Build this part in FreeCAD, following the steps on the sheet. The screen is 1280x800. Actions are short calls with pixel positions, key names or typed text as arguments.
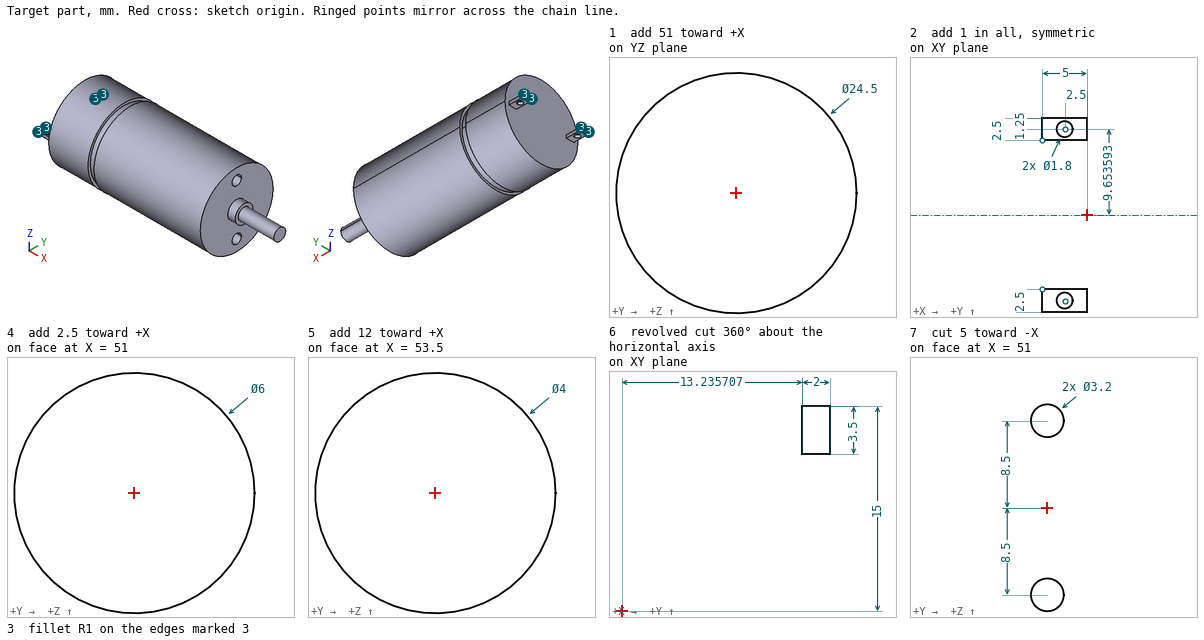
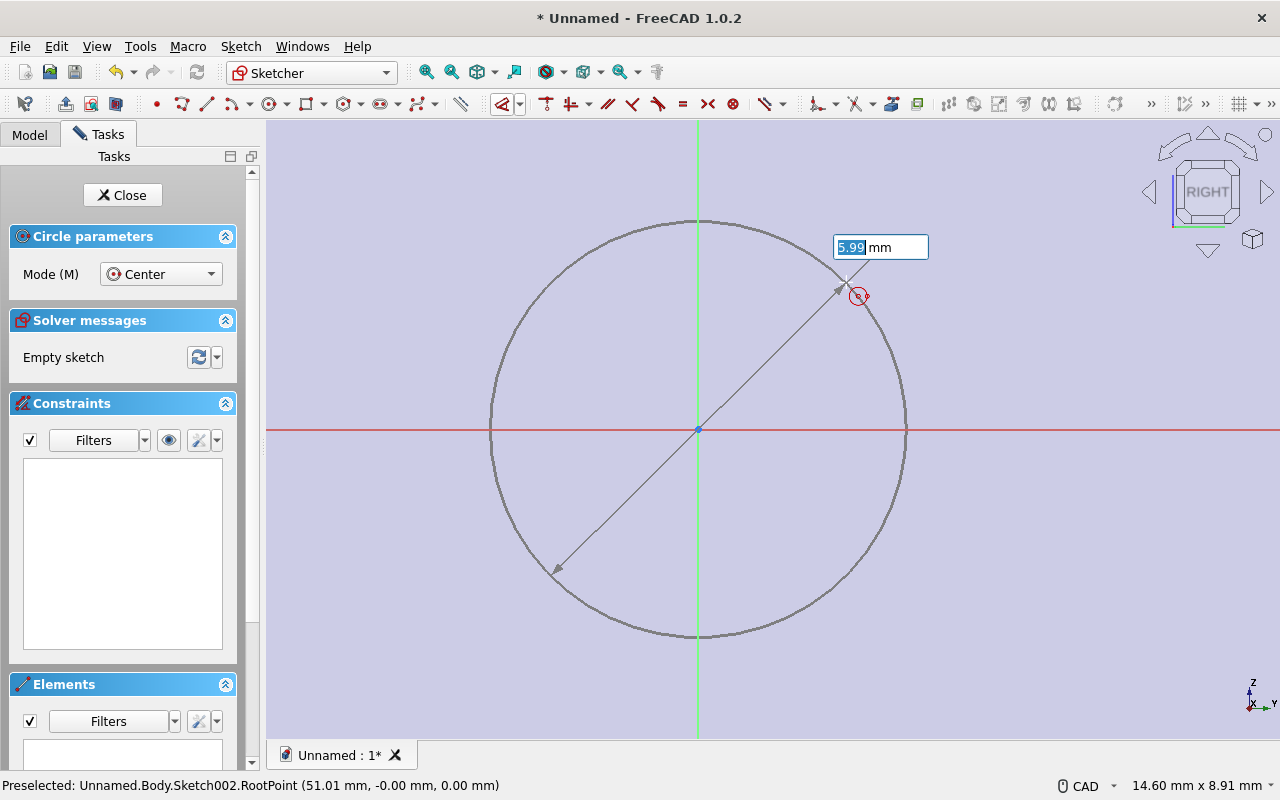
text(6)
key(Return)
key(Escape)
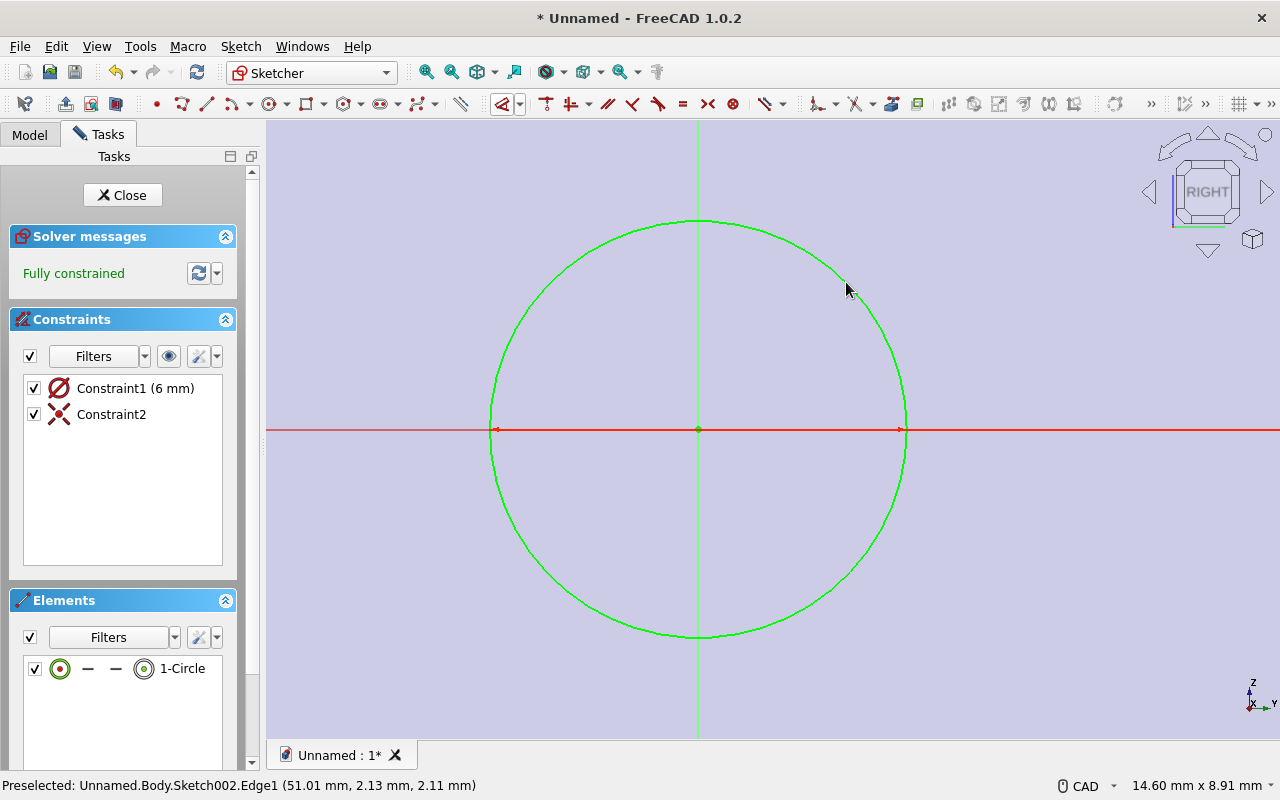
click(123, 195)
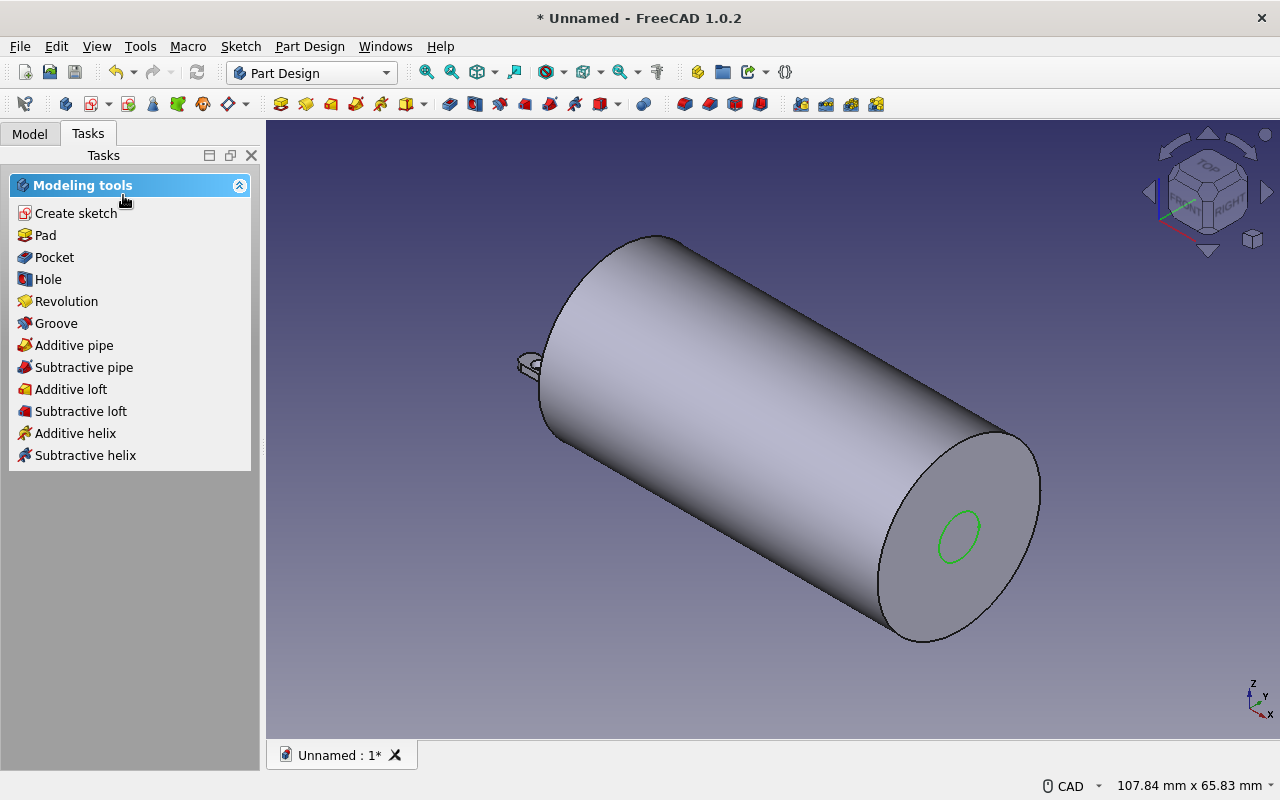
click(281, 104)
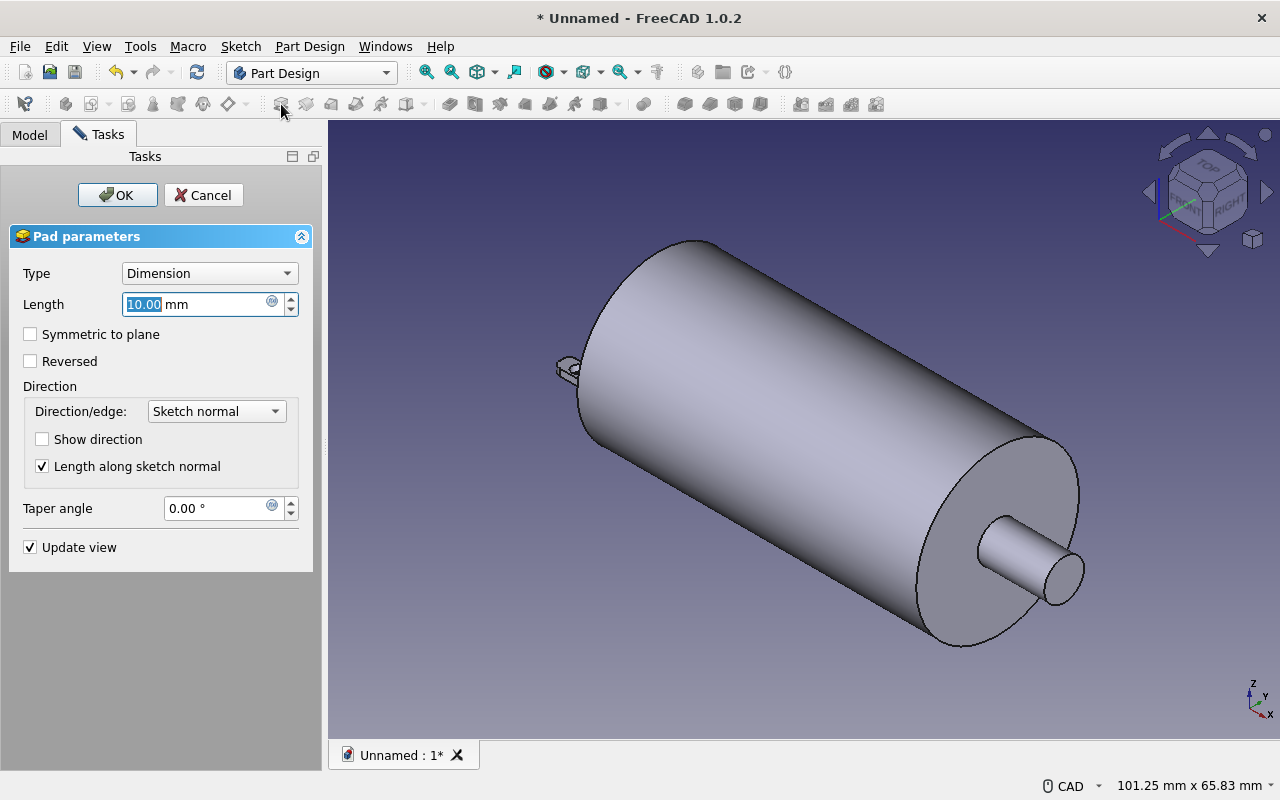
text(2.5)
key(Tab)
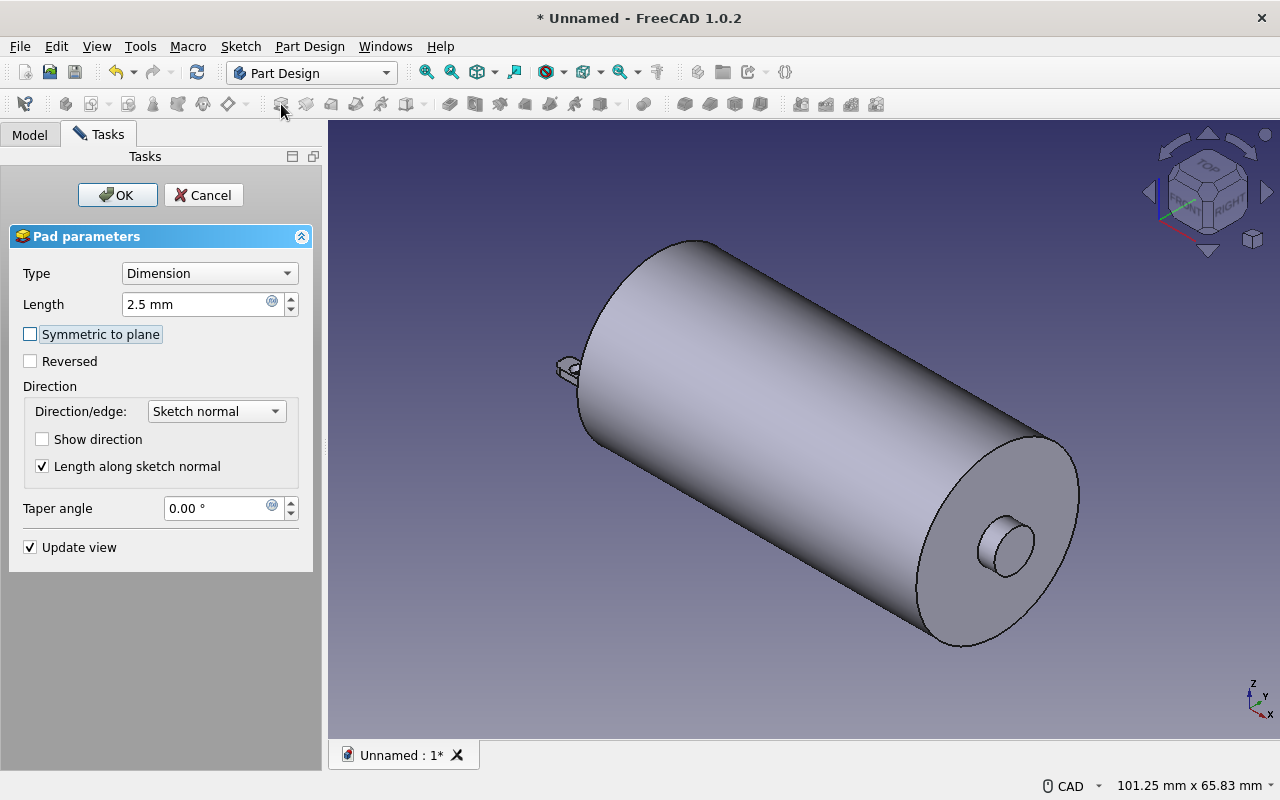
click(118, 195)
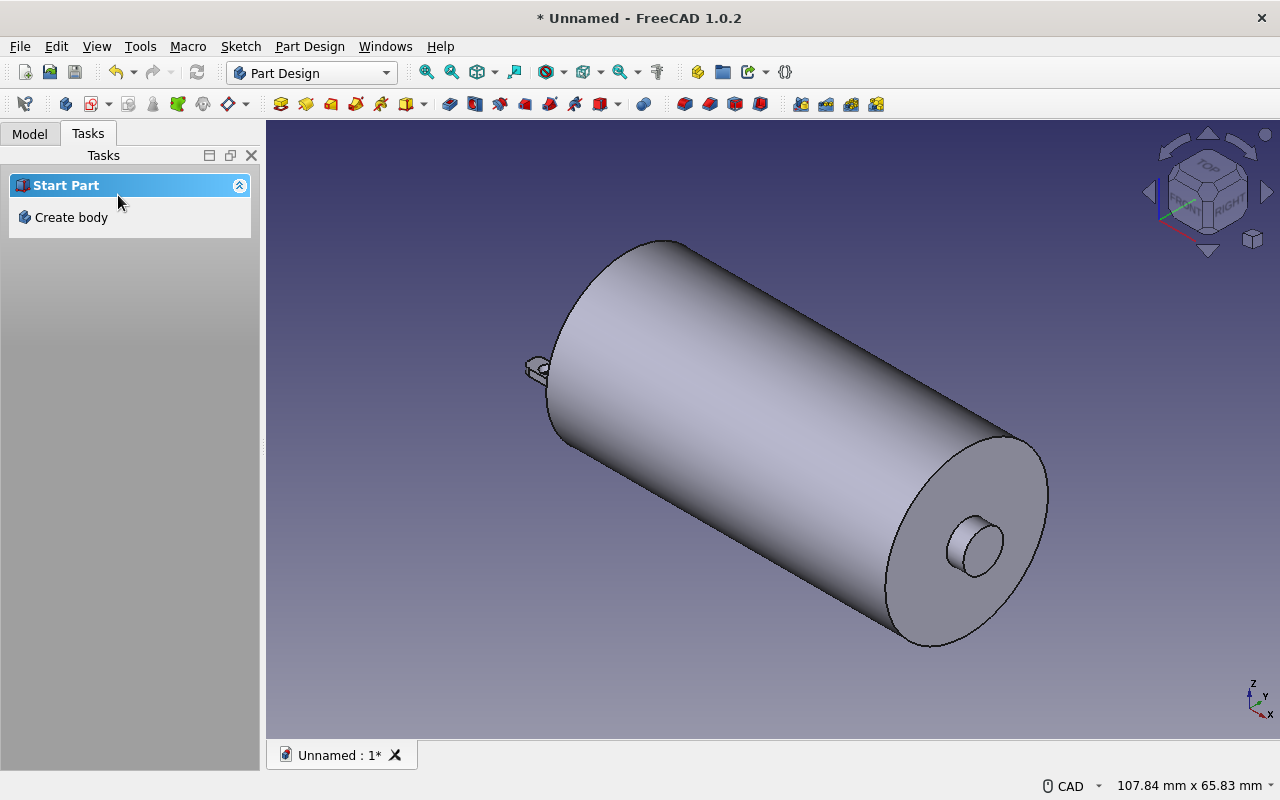
click(983, 550)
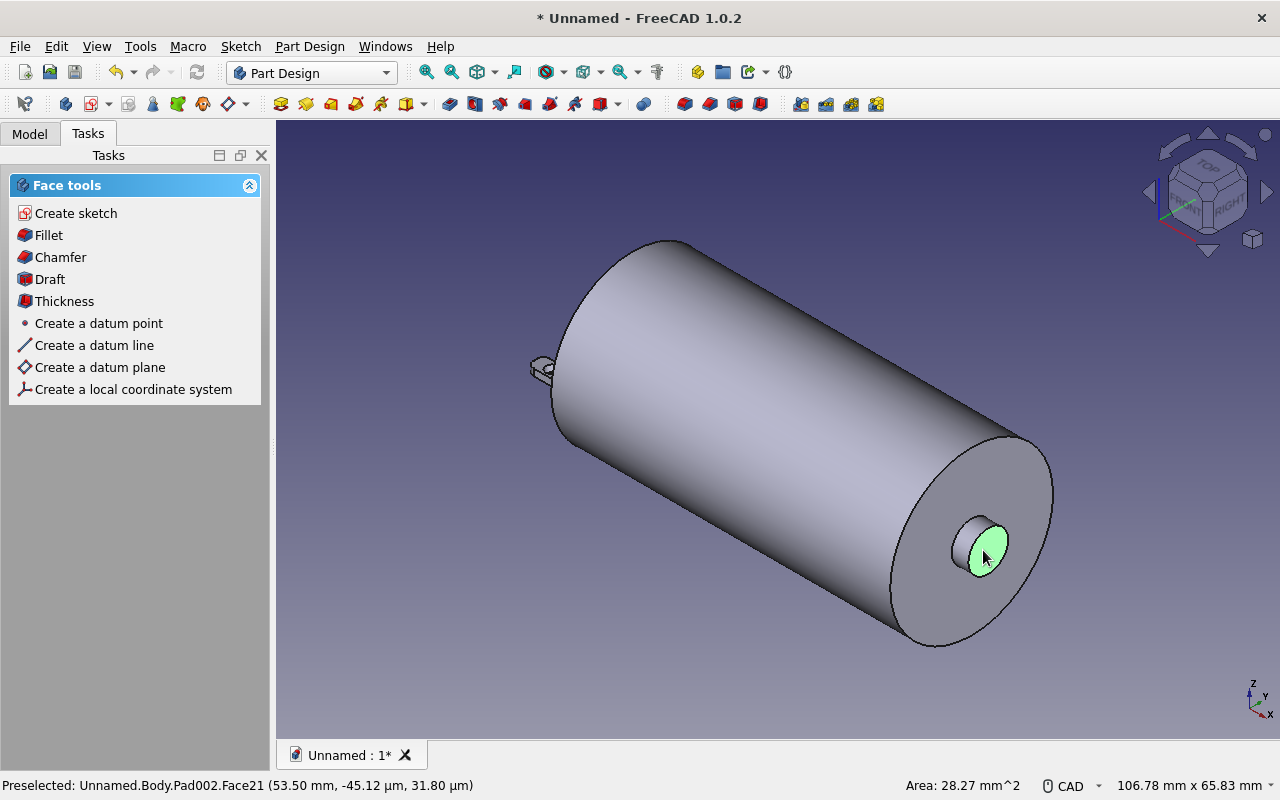
click(90, 104)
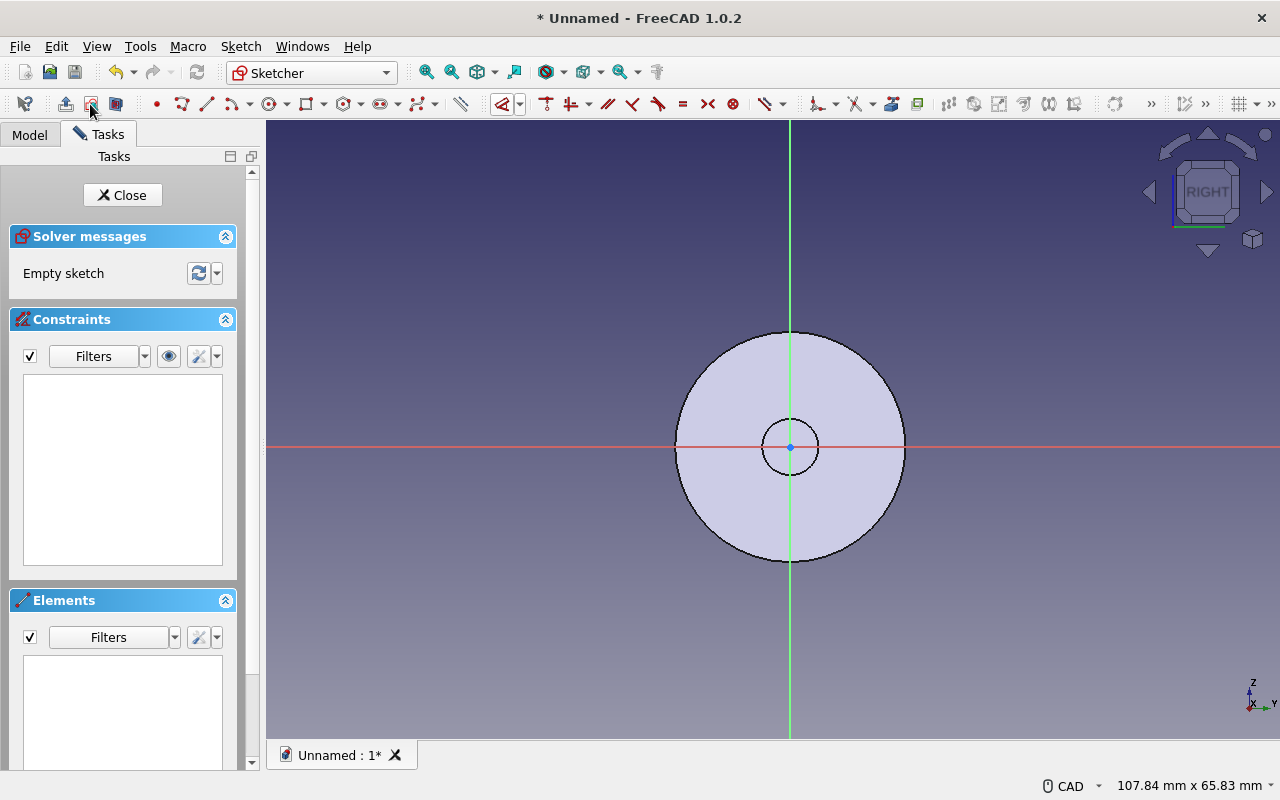
scroll(799, 449, up, 12)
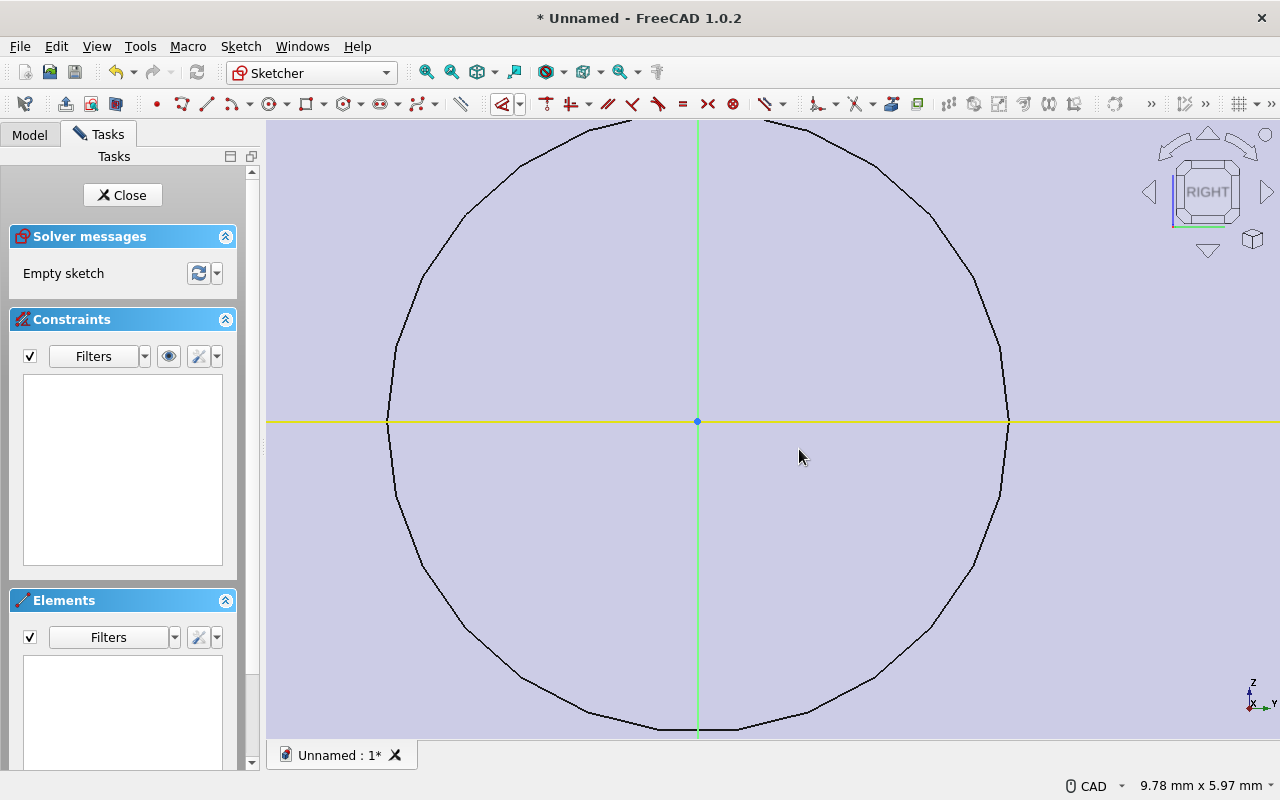
click(268, 104)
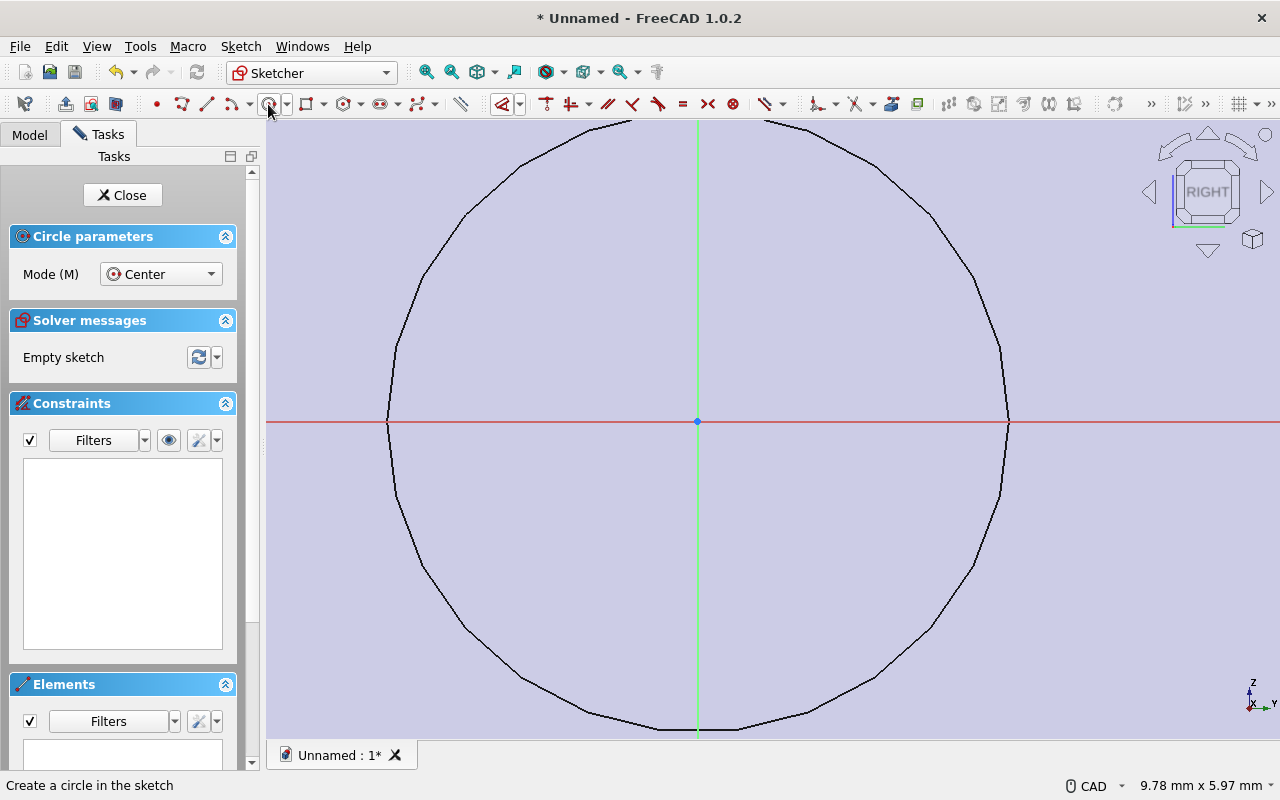
click(698, 422)
move(845, 275)